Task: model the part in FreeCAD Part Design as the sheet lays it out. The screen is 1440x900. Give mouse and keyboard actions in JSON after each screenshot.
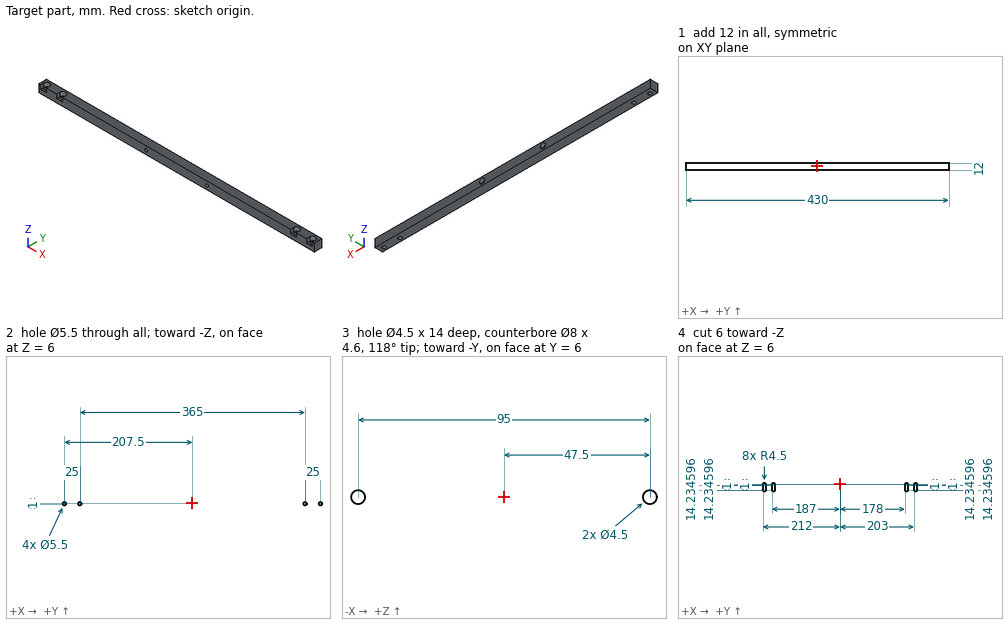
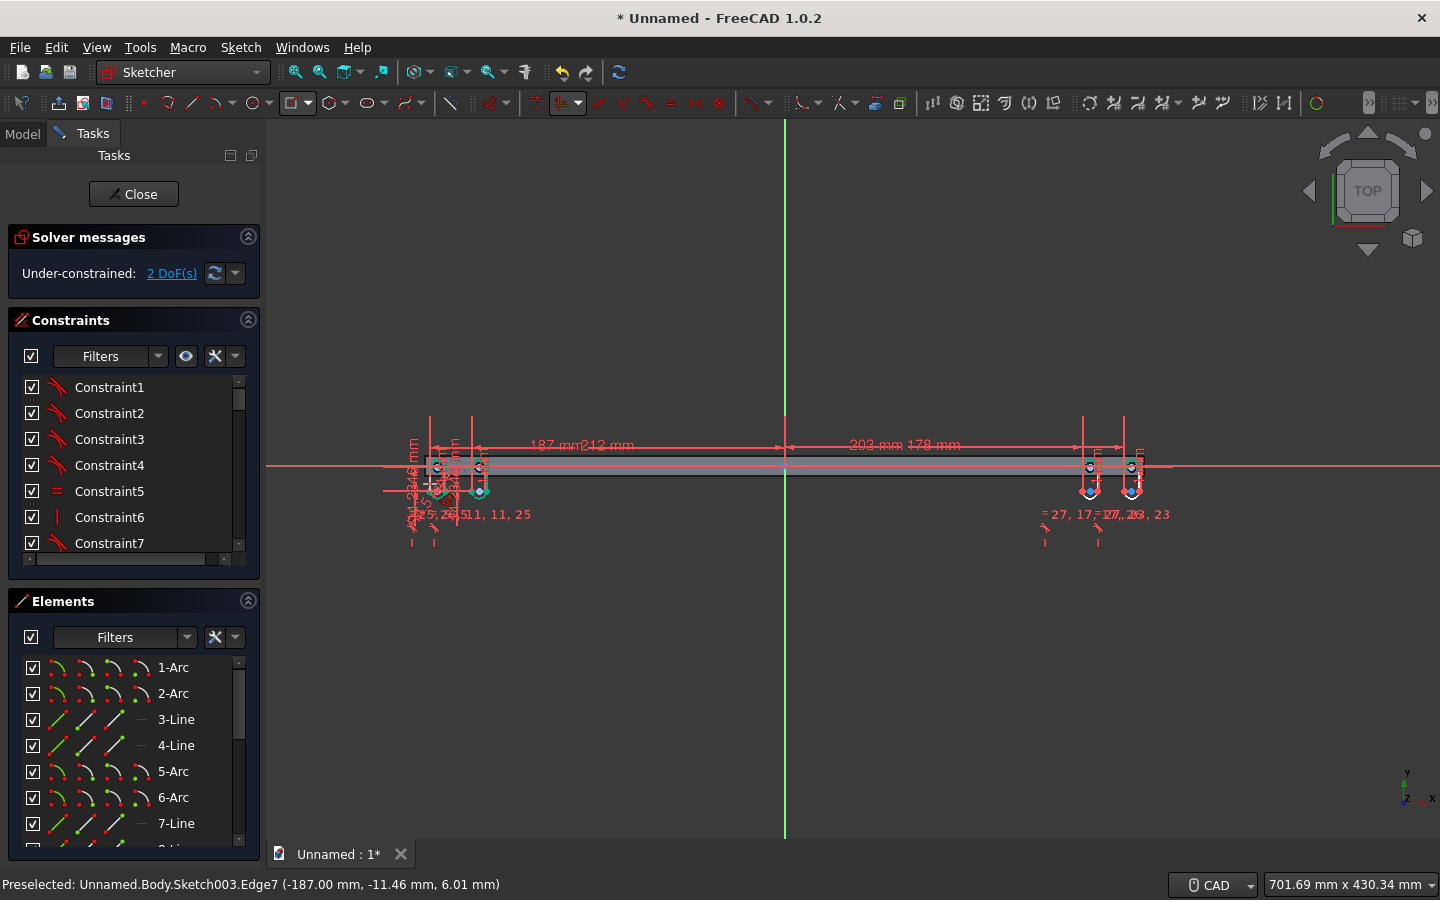
{"action": "scroll", "coordinate": [1083, 484], "scroll_direction": "up", "scroll_amount": 4}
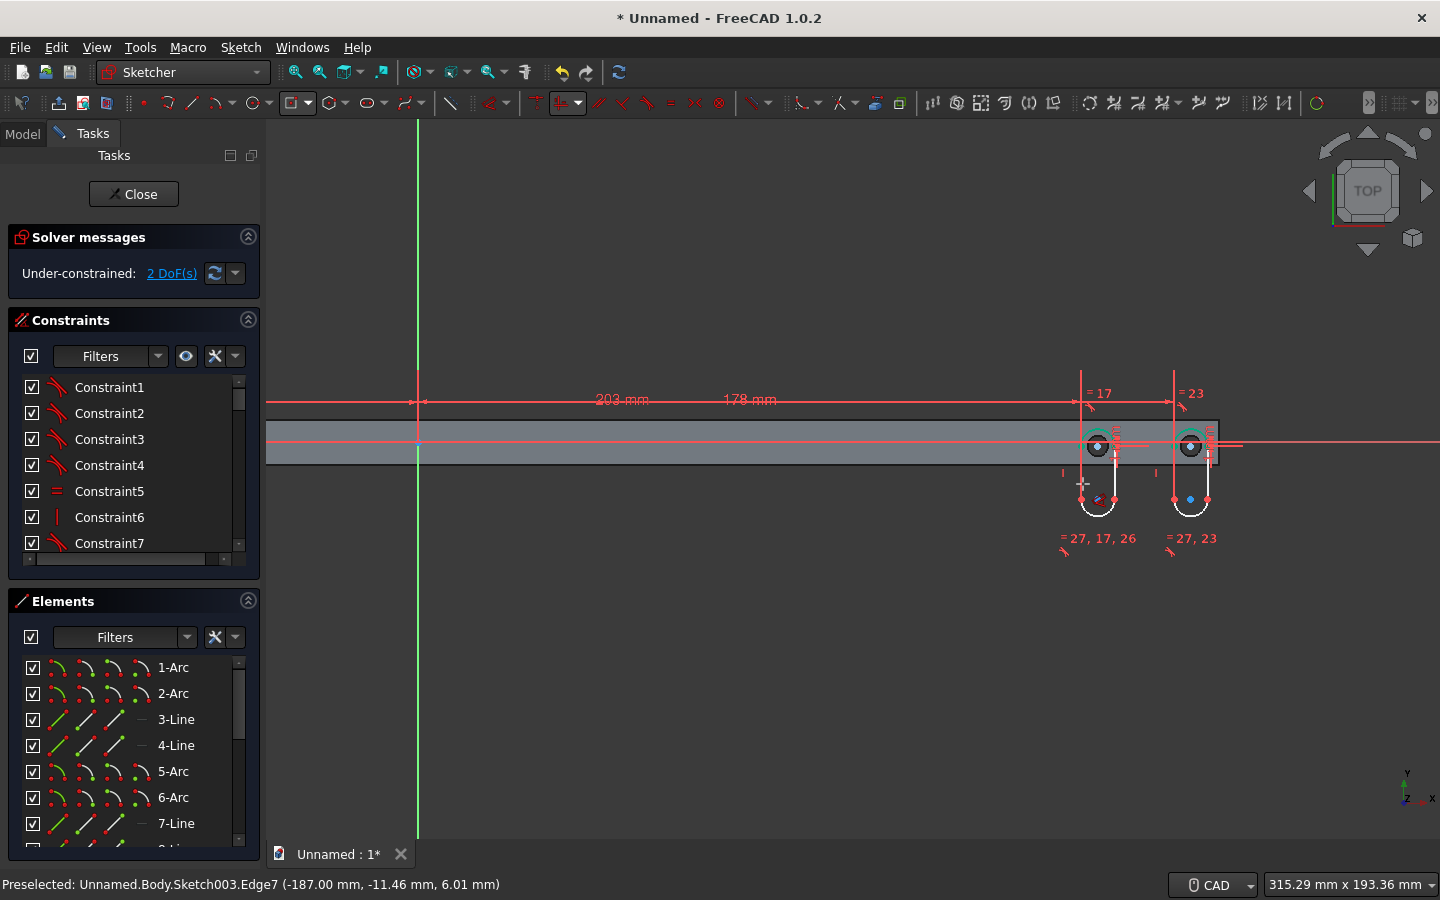
{"action": "left_click", "coordinate": [1081, 483]}
{"action": "left_click", "coordinate": [1047, 473]}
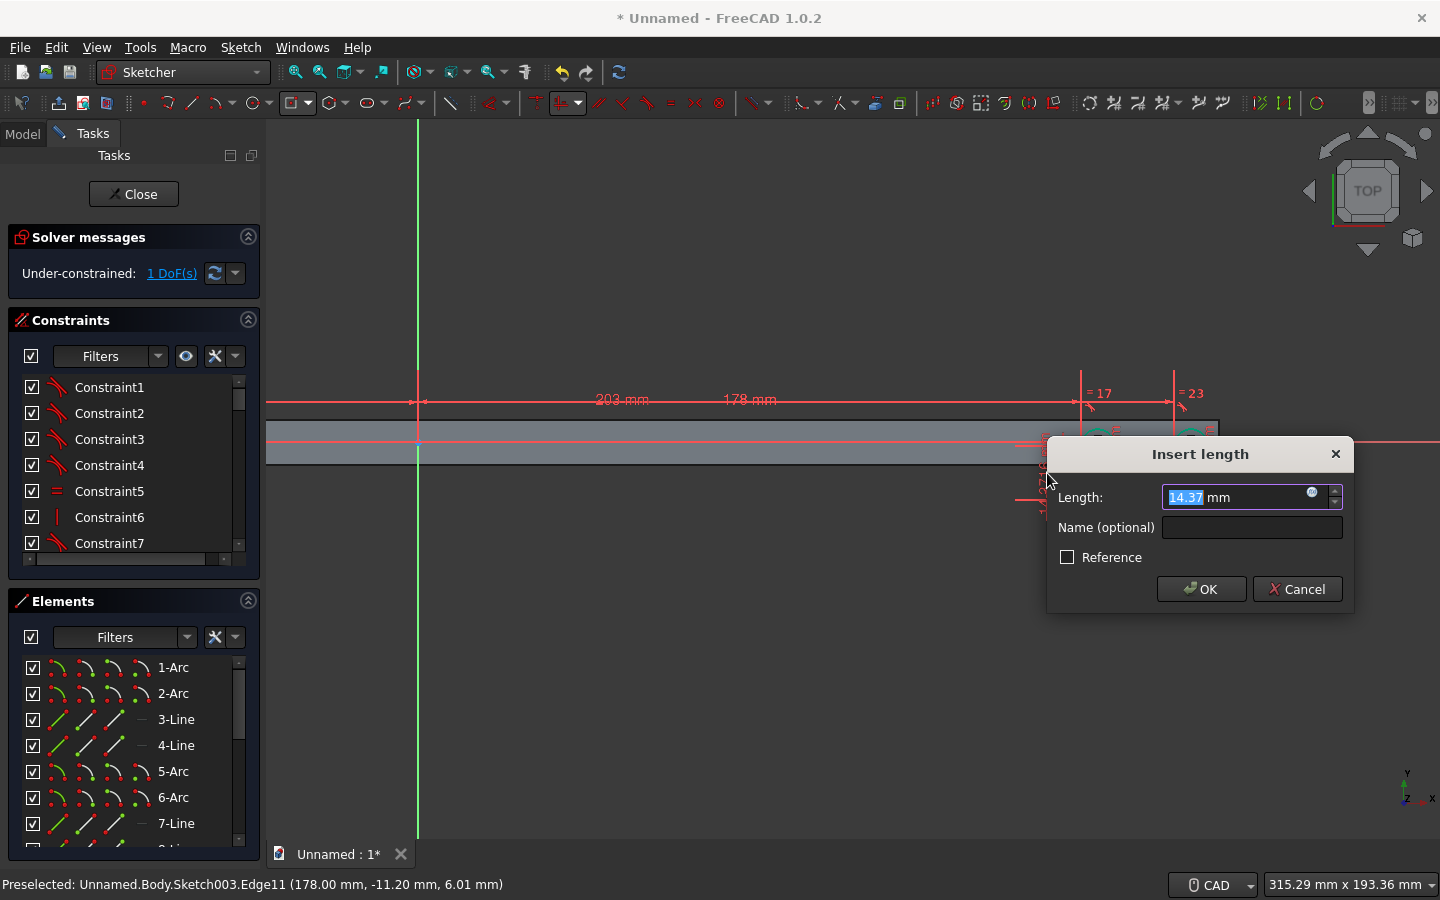
{"action": "type", "text": "14.234596"}
{"action": "key", "text": "Return"}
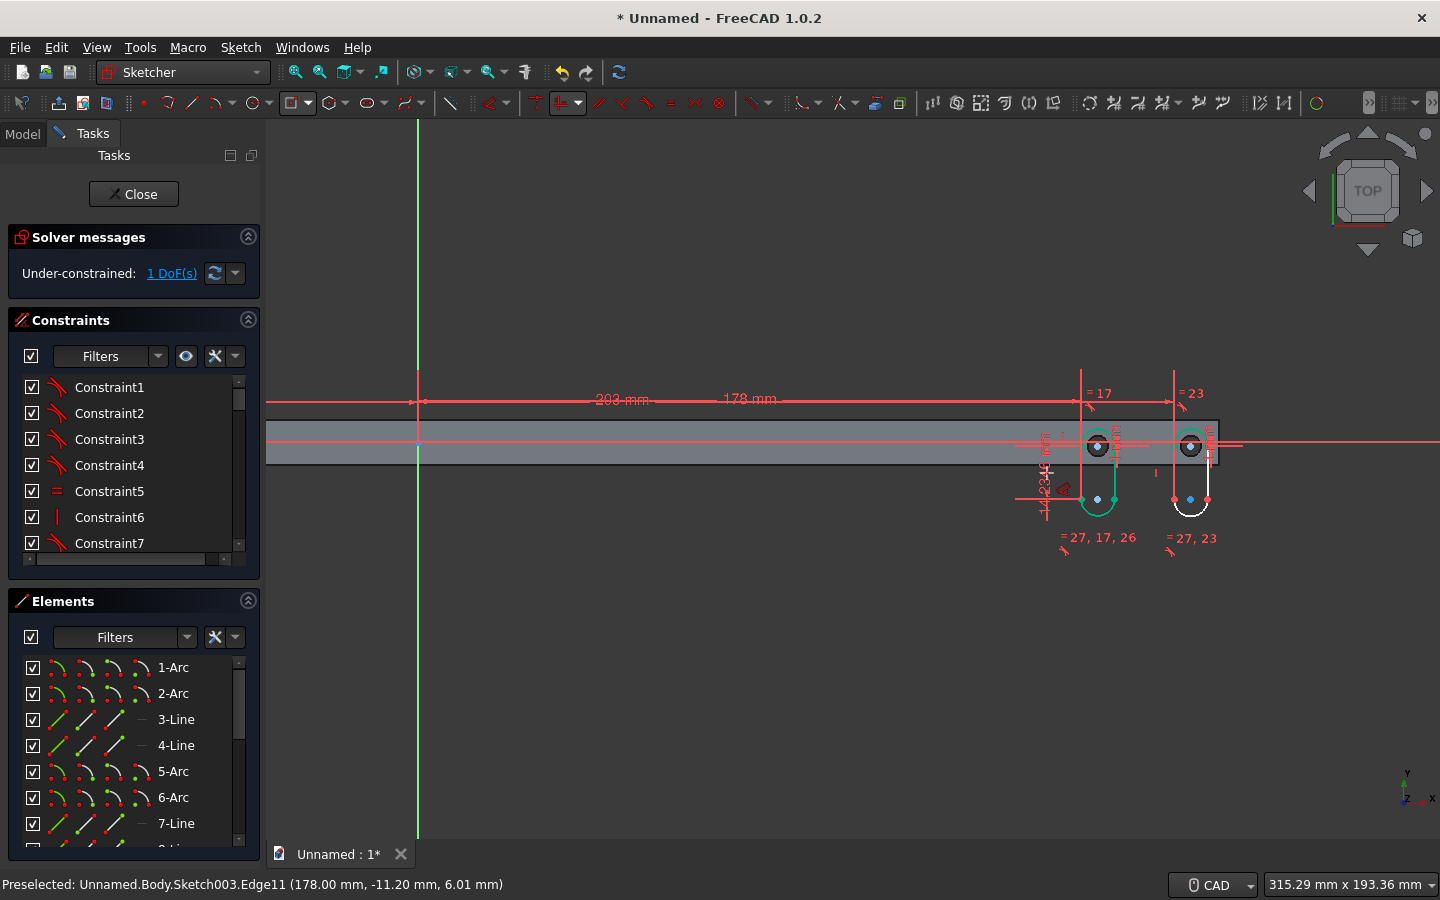
{"action": "left_click", "coordinate": [1174, 484]}
{"action": "left_click", "coordinate": [1140, 473]}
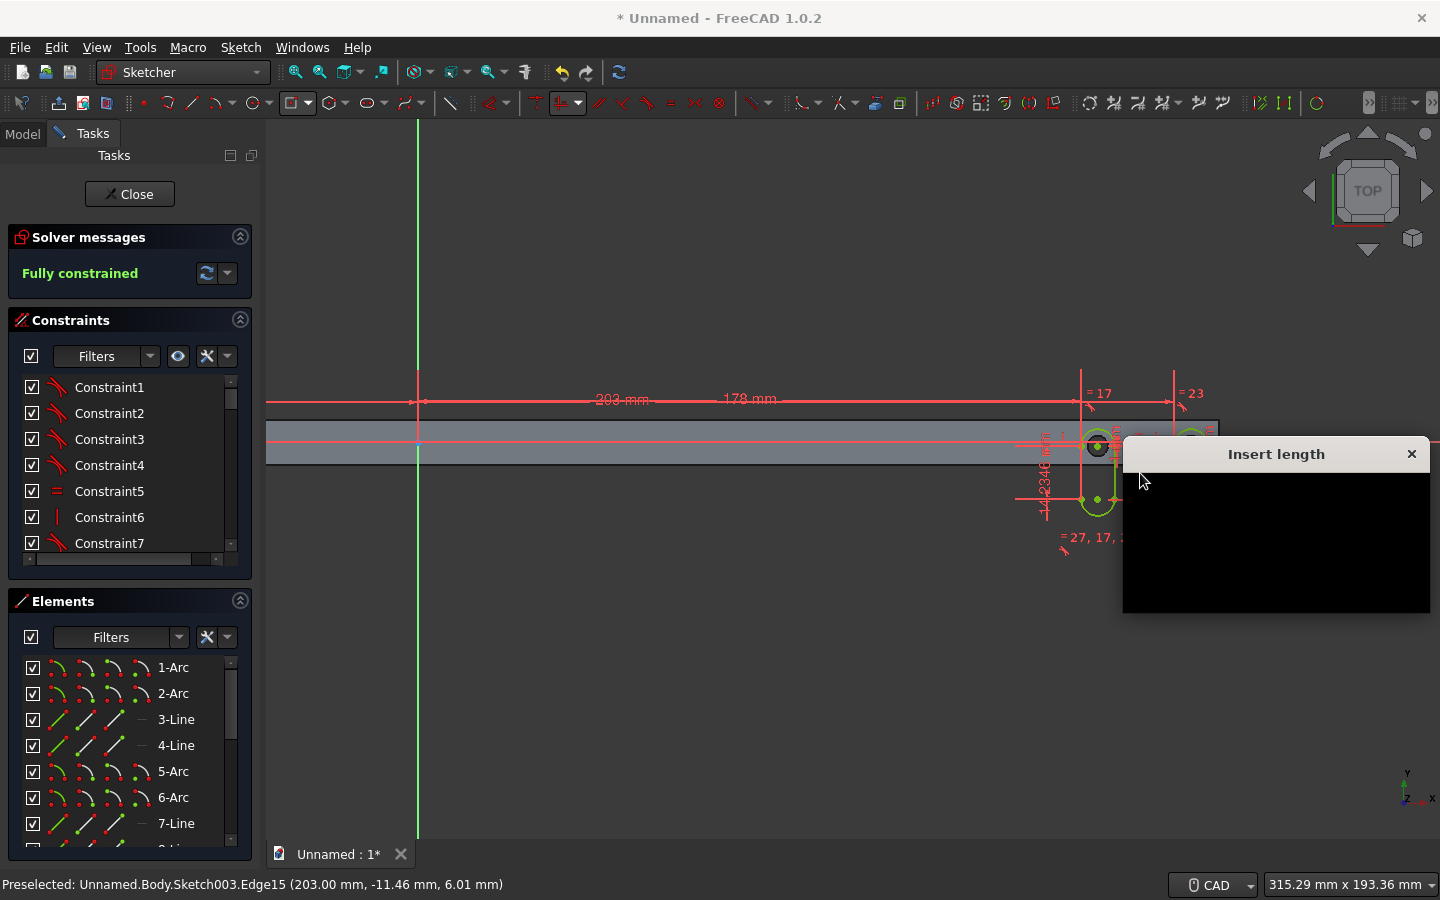
{"action": "type", "text": "14.234596"}
{"action": "key", "text": "Return"}
{"action": "key", "text": "Escape"}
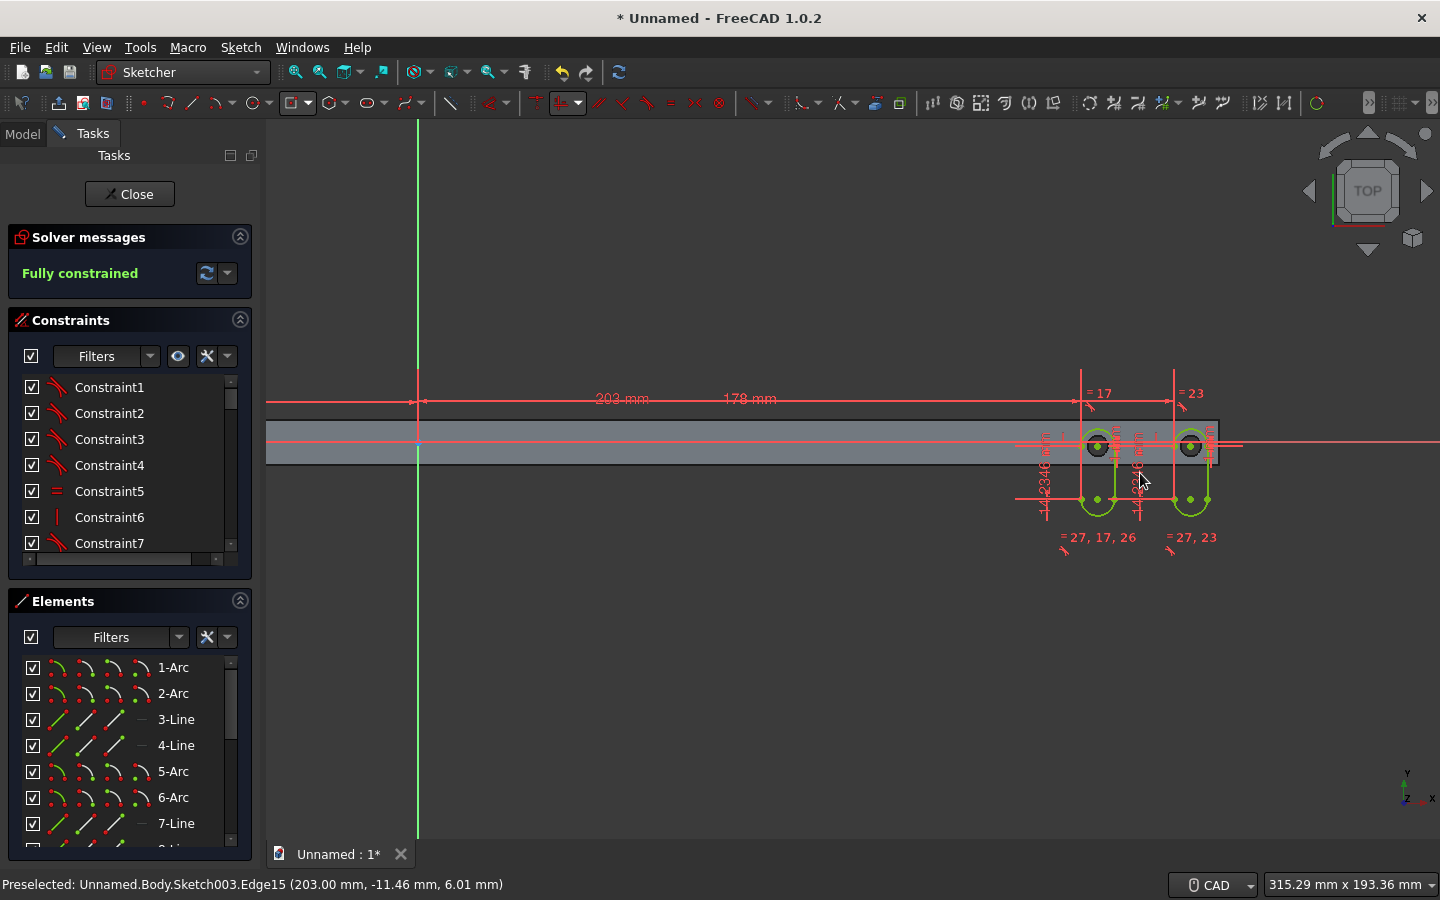
{"action": "left_click", "coordinate": [130, 194]}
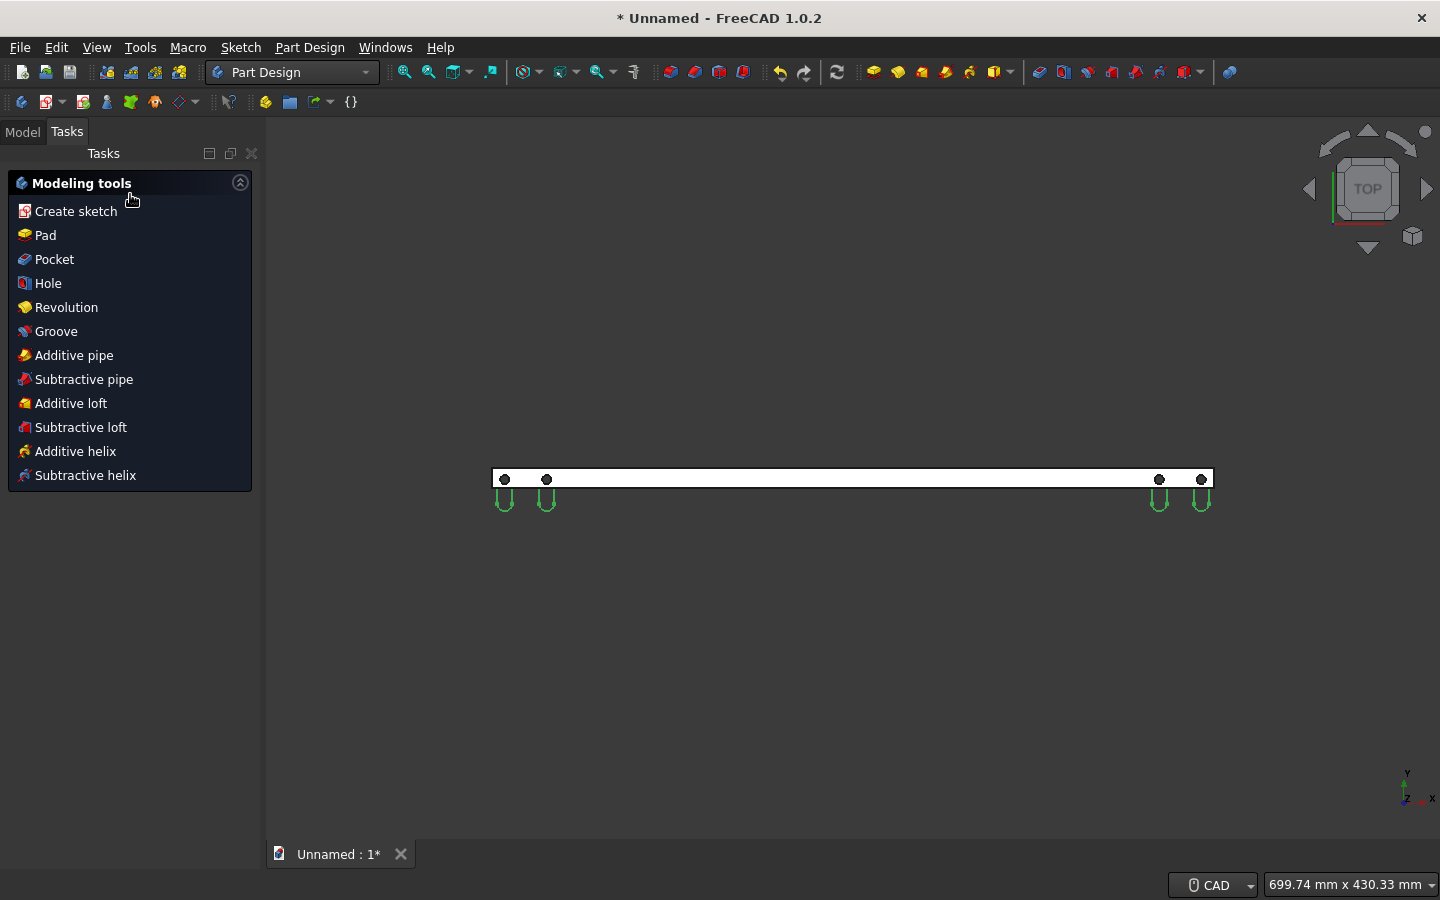
{"action": "left_click", "coordinate": [1040, 72]}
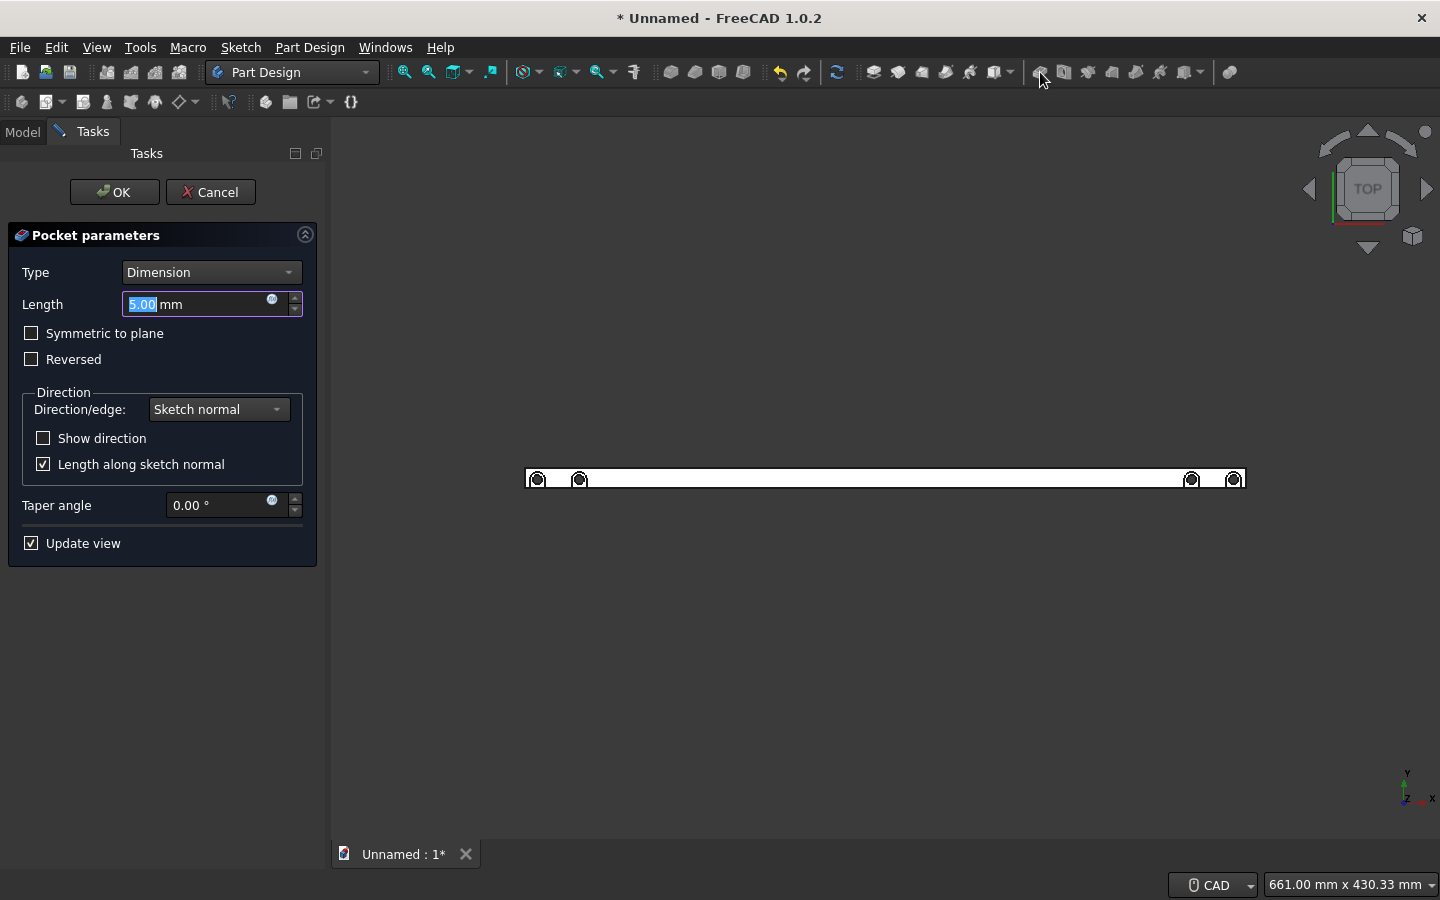
{"action": "type", "text": "6"}
{"action": "key", "text": "Tab"}